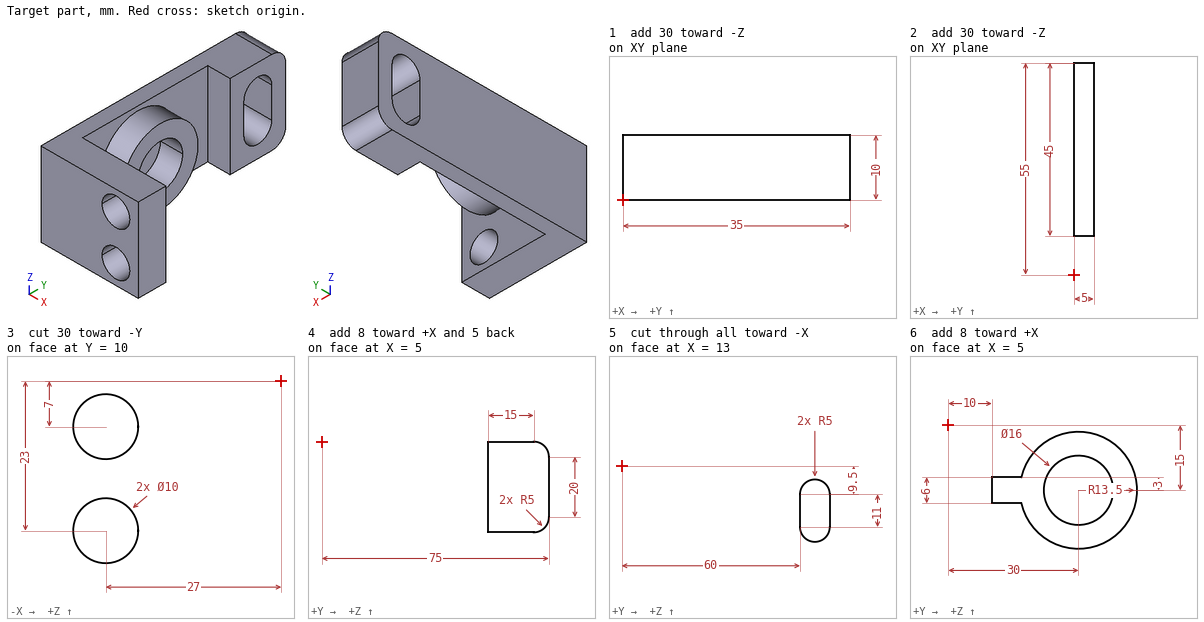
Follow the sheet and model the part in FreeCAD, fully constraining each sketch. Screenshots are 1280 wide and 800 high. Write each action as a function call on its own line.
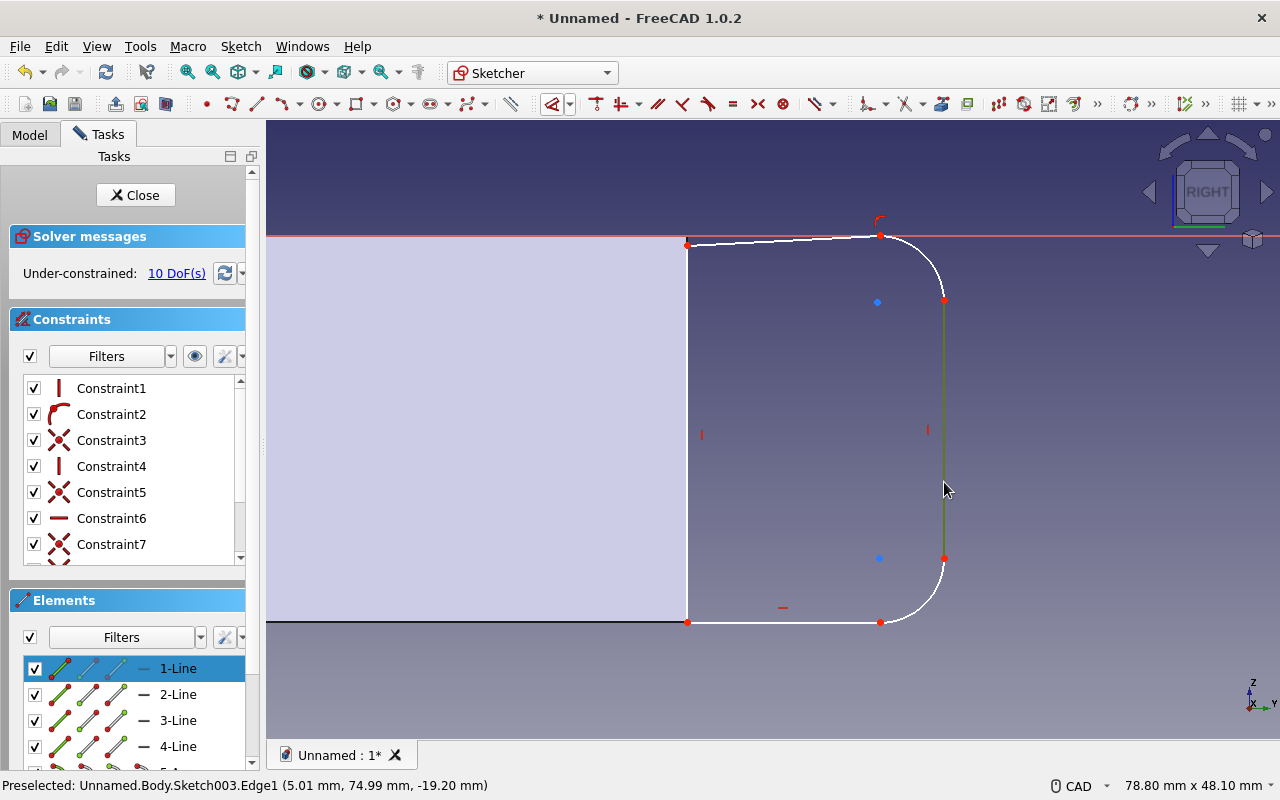
click(937, 272)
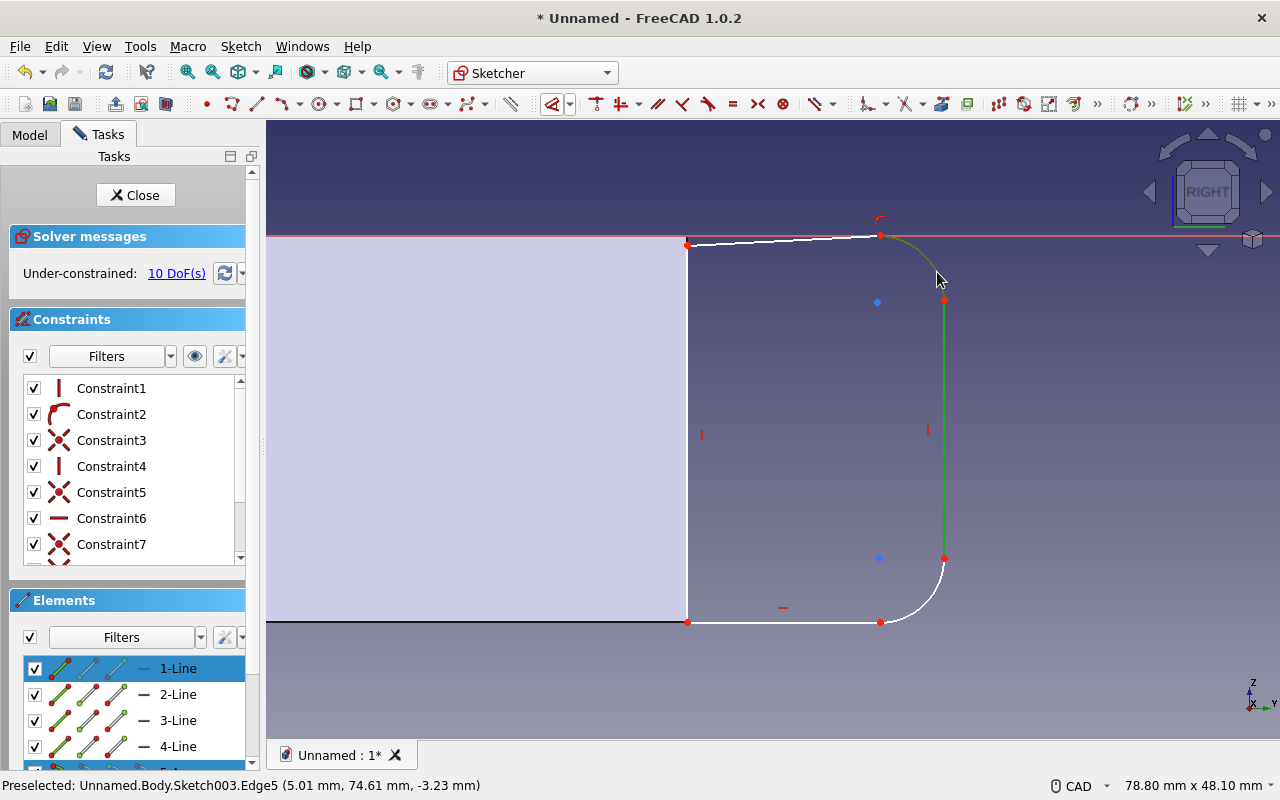
key(t)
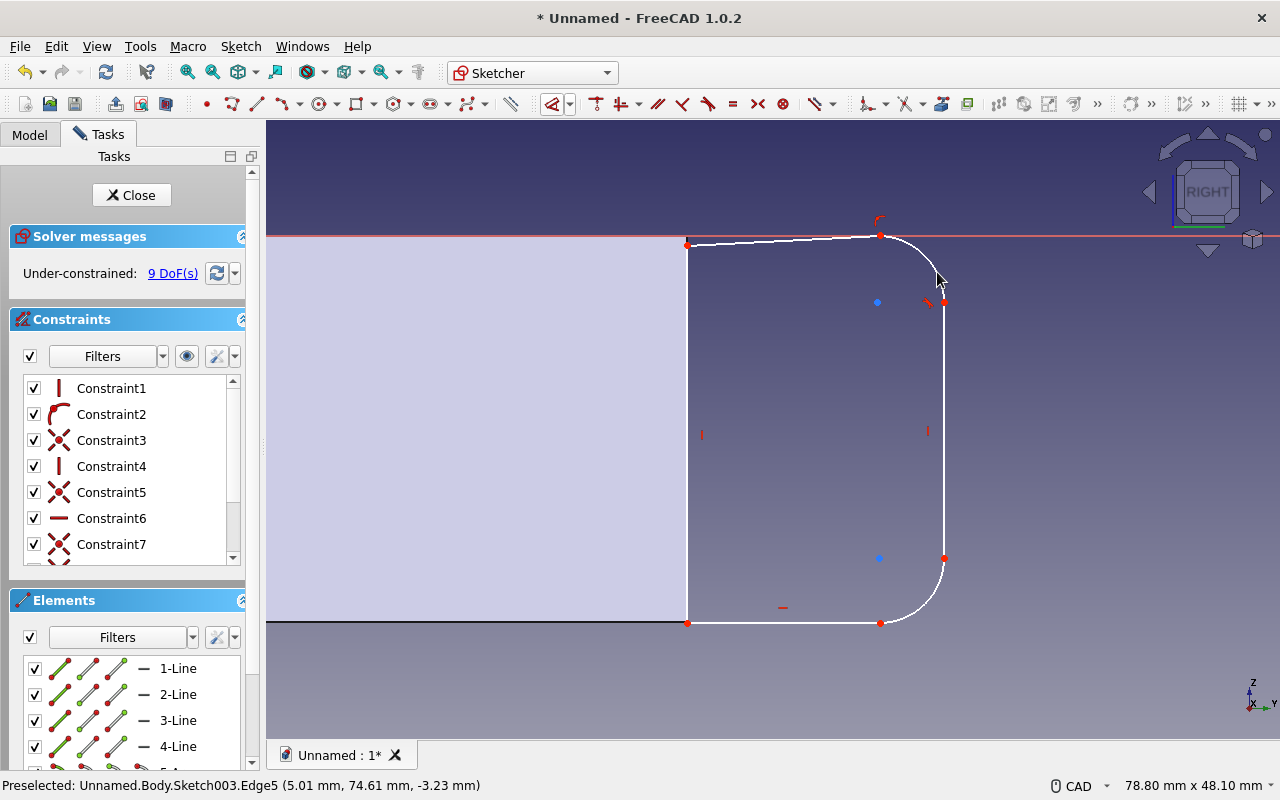
click(944, 482)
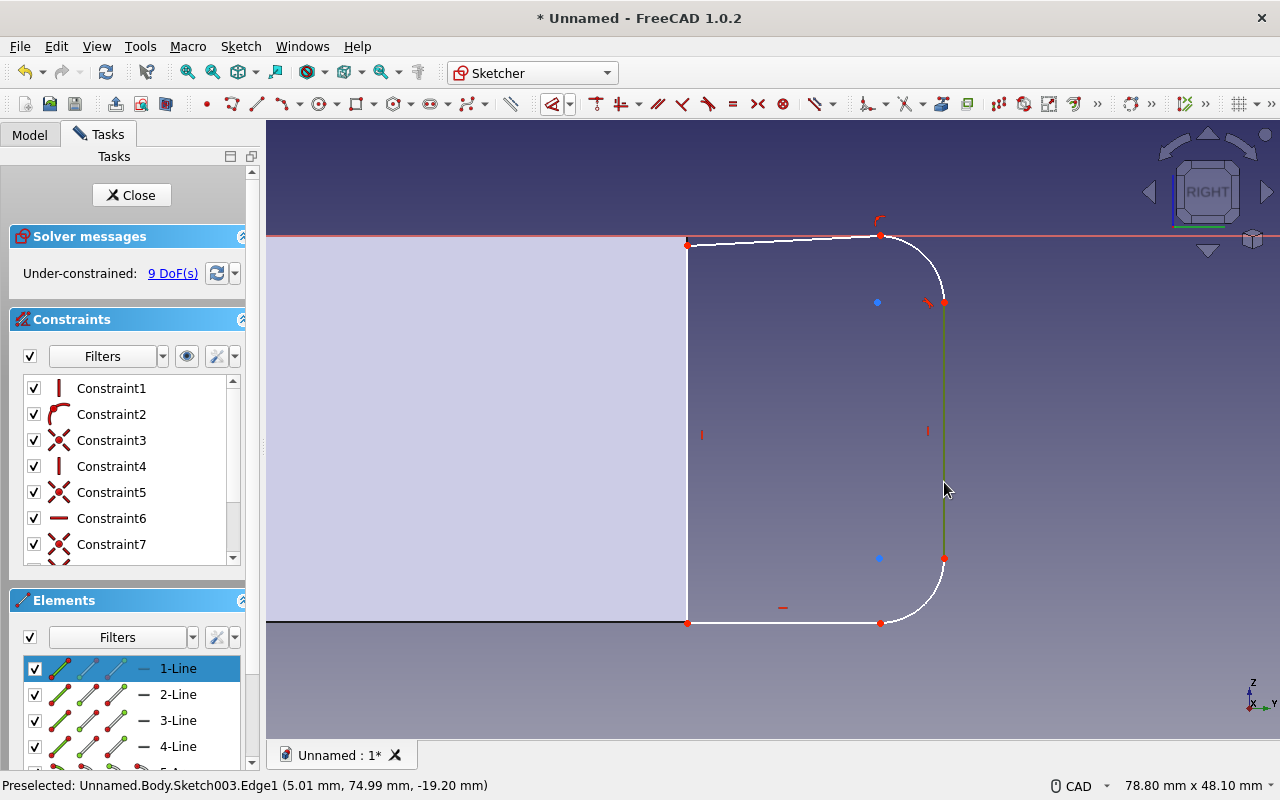
click(909, 616)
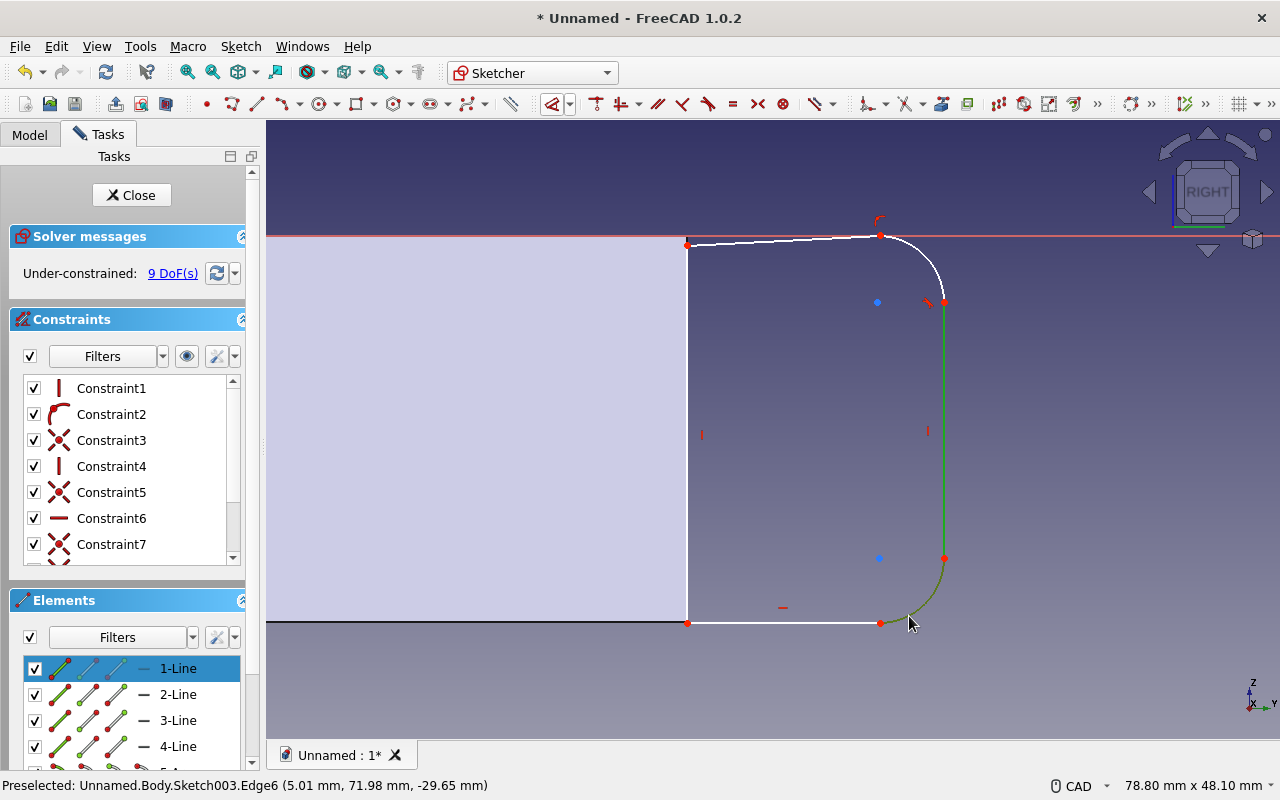
click(708, 104)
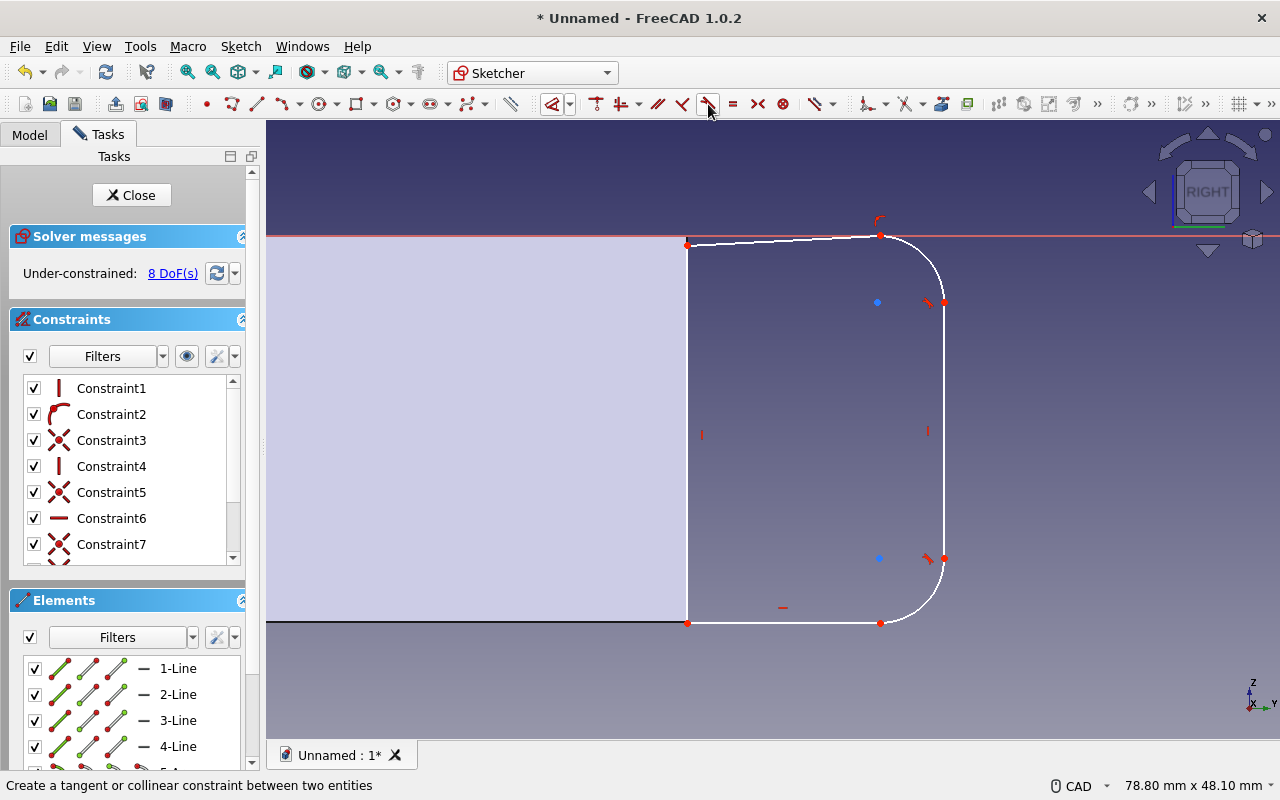
click(822, 239)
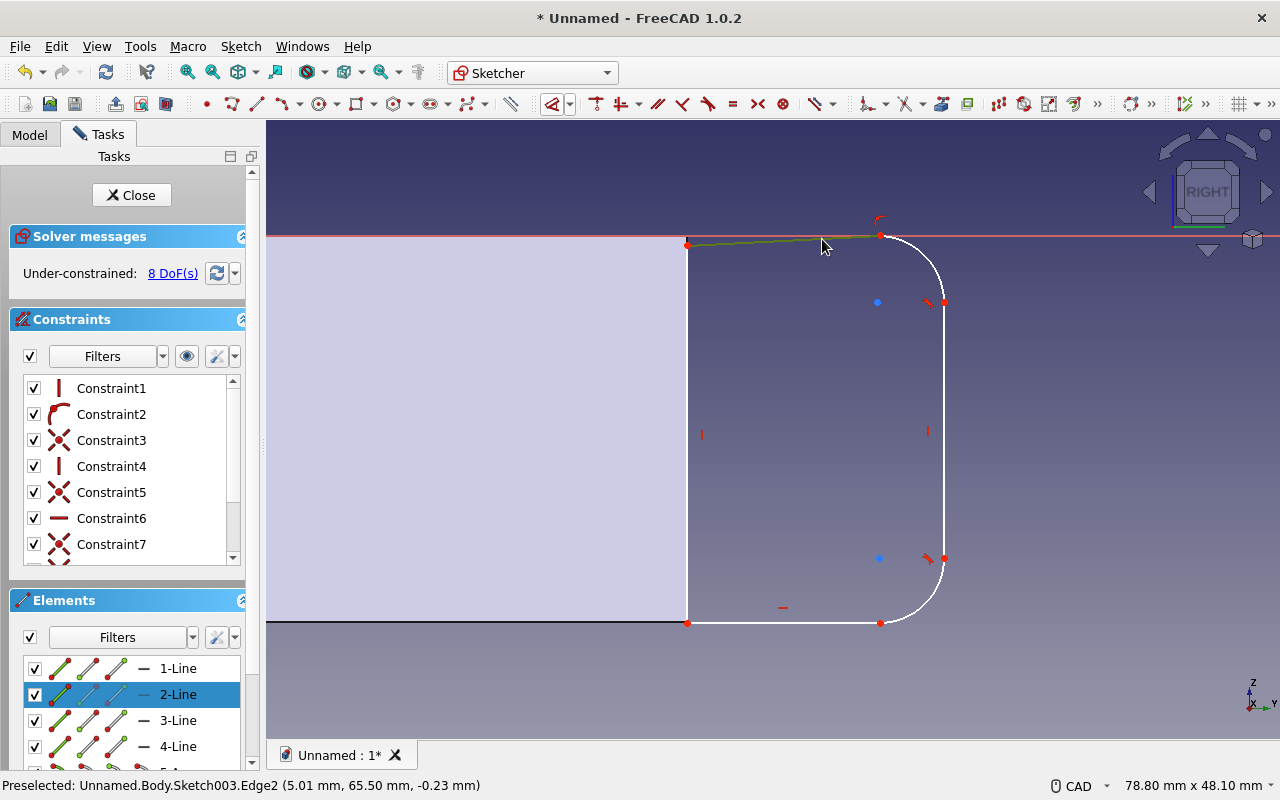
click(937, 273)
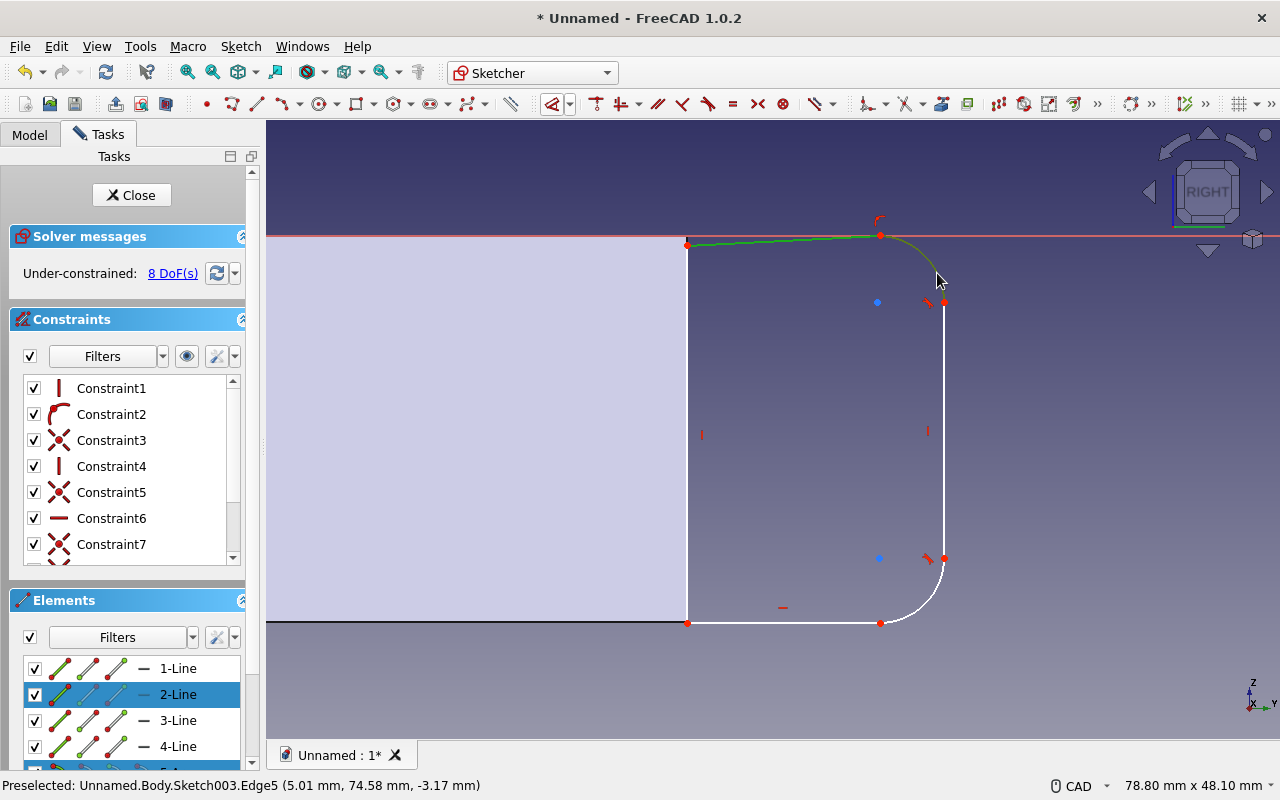
key(t)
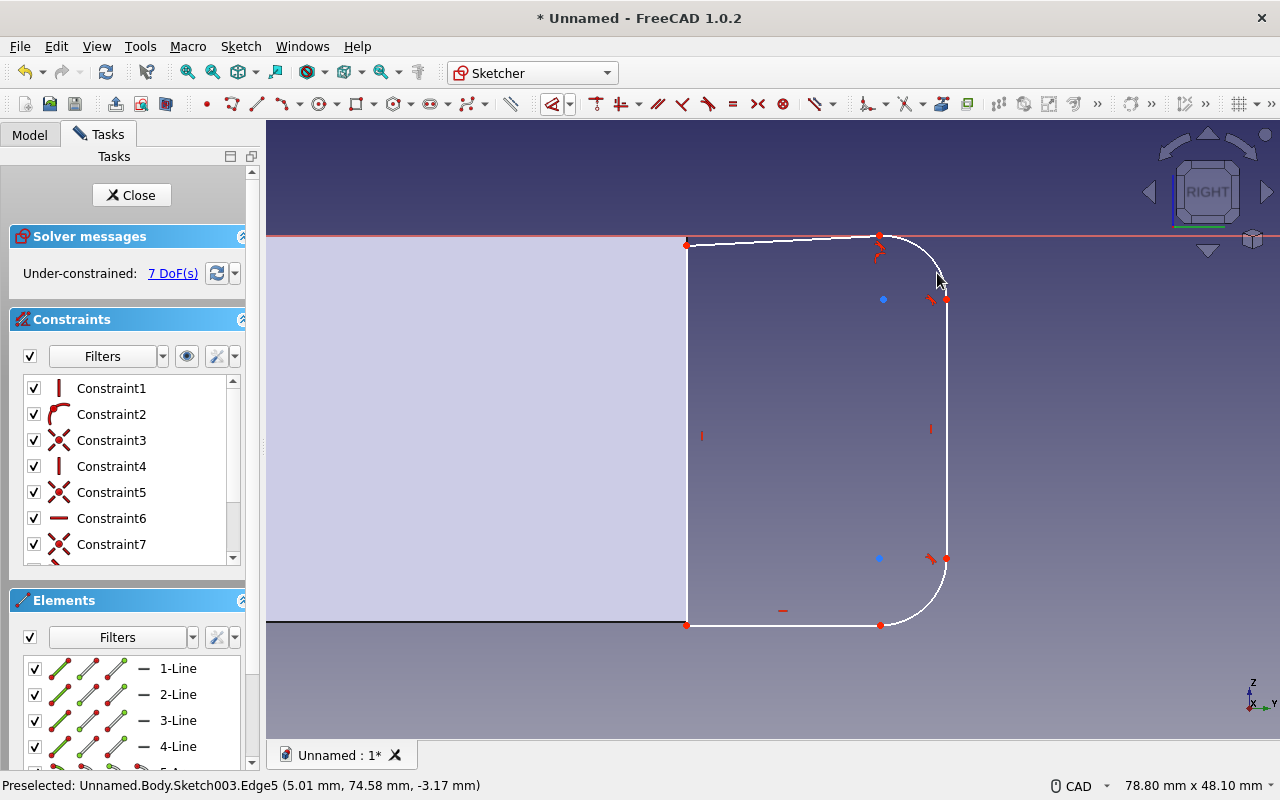
click(745, 626)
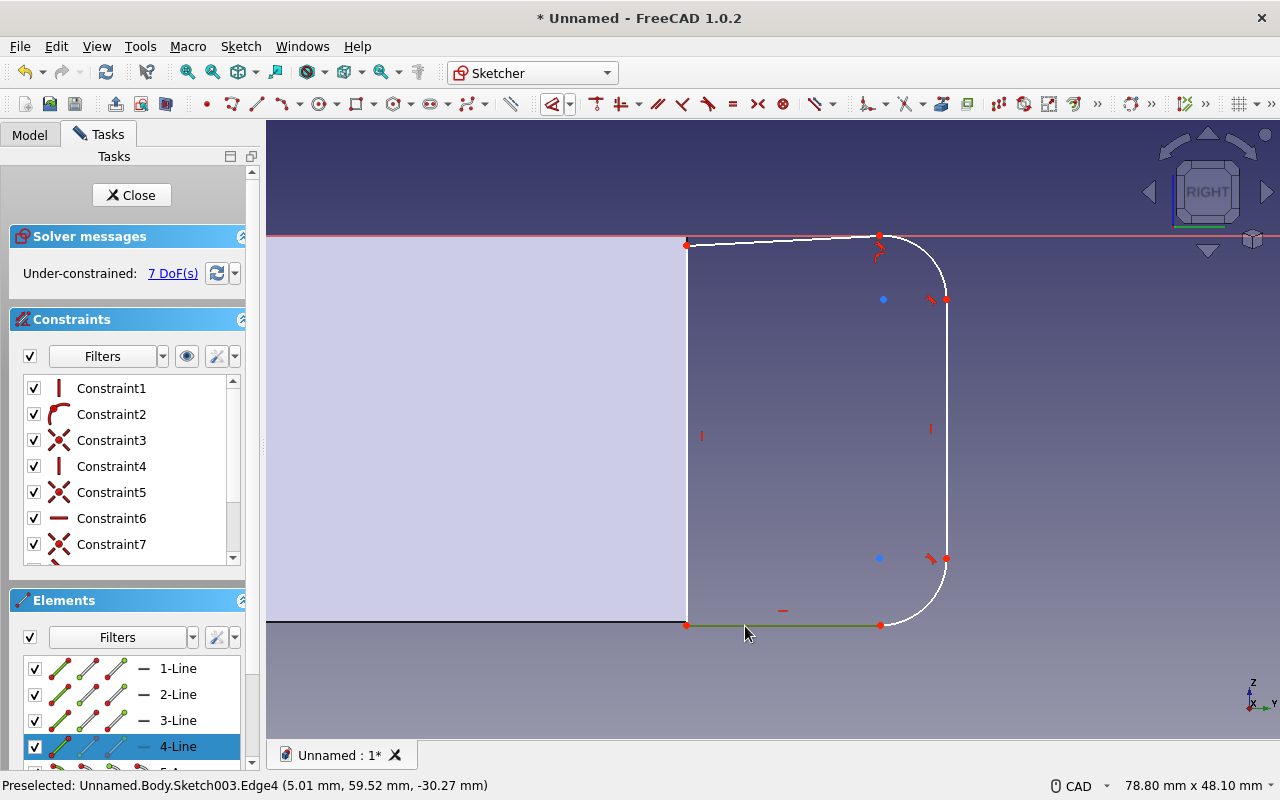
click(910, 618)